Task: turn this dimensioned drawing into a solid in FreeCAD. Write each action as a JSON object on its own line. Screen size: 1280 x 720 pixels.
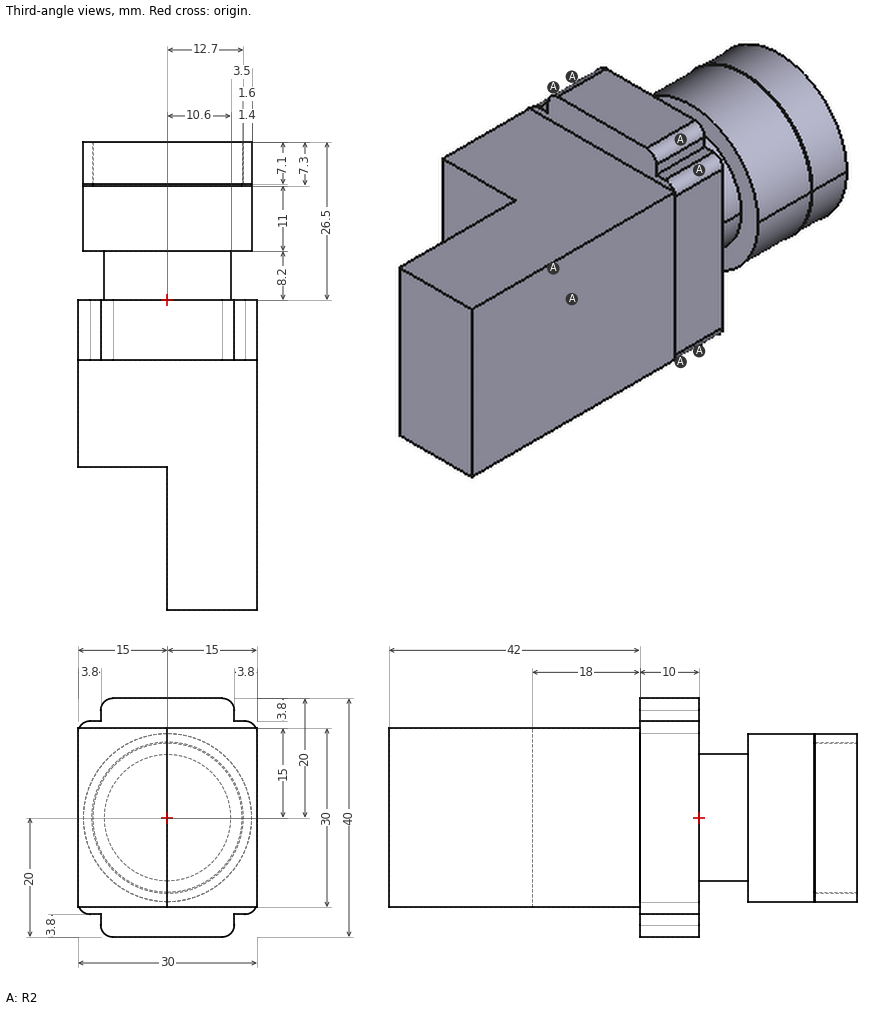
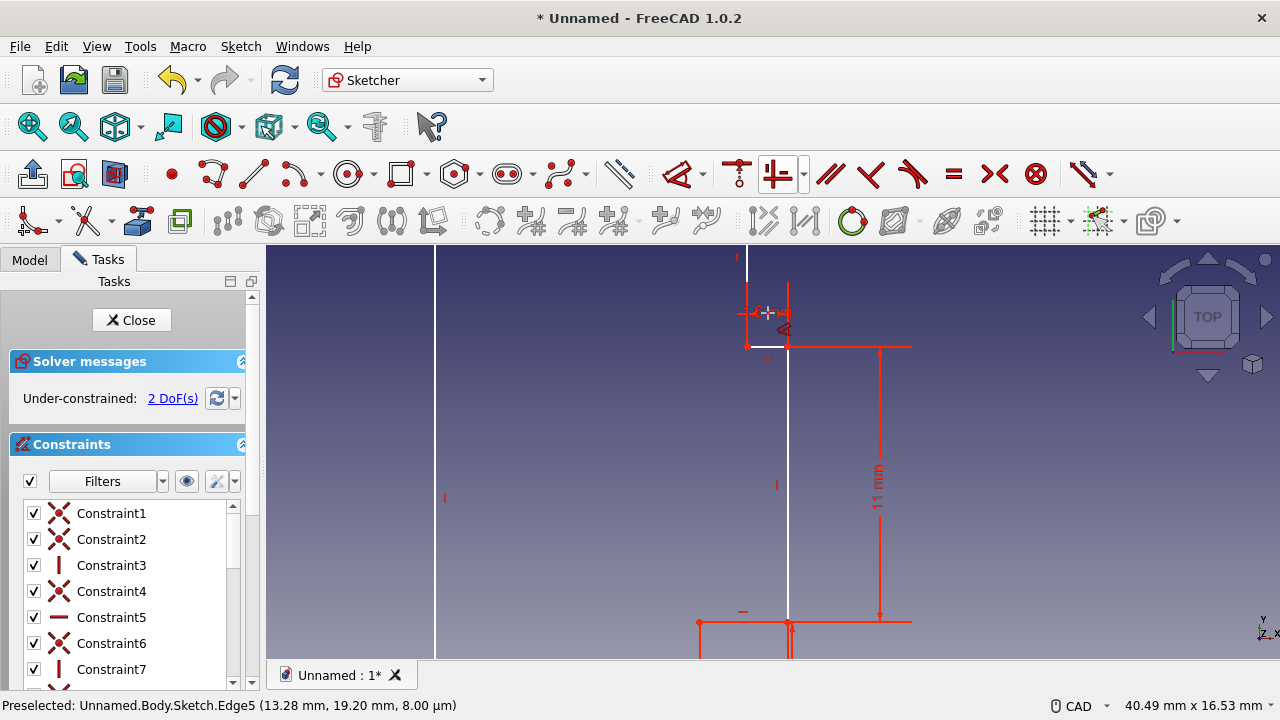
{"action": "left_click", "coordinate": [747, 293]}
{"action": "left_click", "coordinate": [781, 284]}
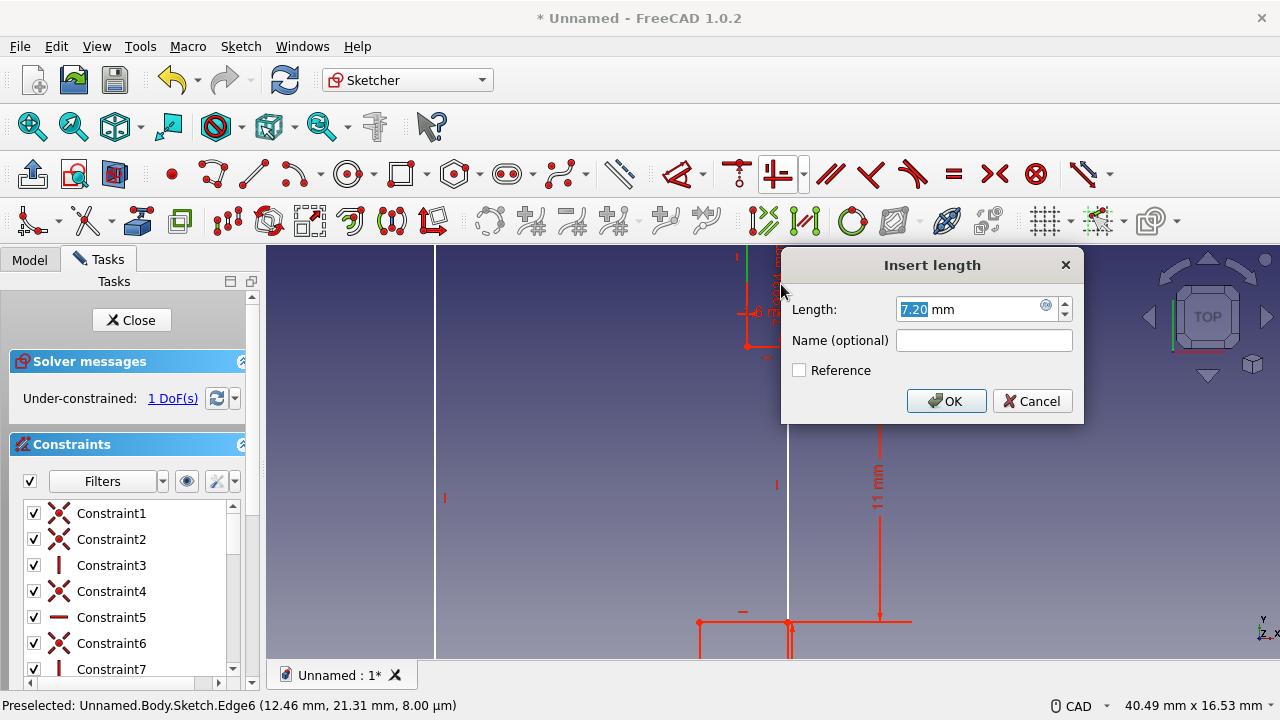
{"action": "type", "text": "7.3"}
{"action": "key", "text": "Return"}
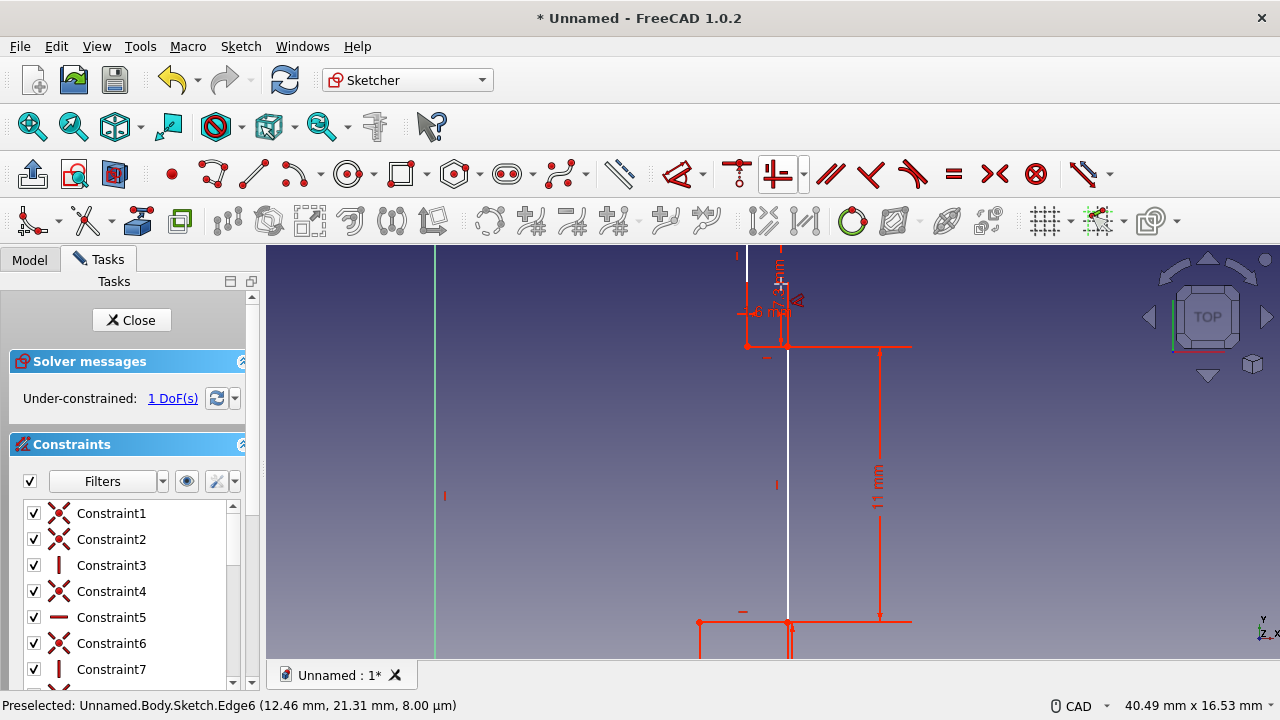
{"action": "scroll", "coordinate": [758, 426], "scroll_direction": "down", "scroll_amount": 5}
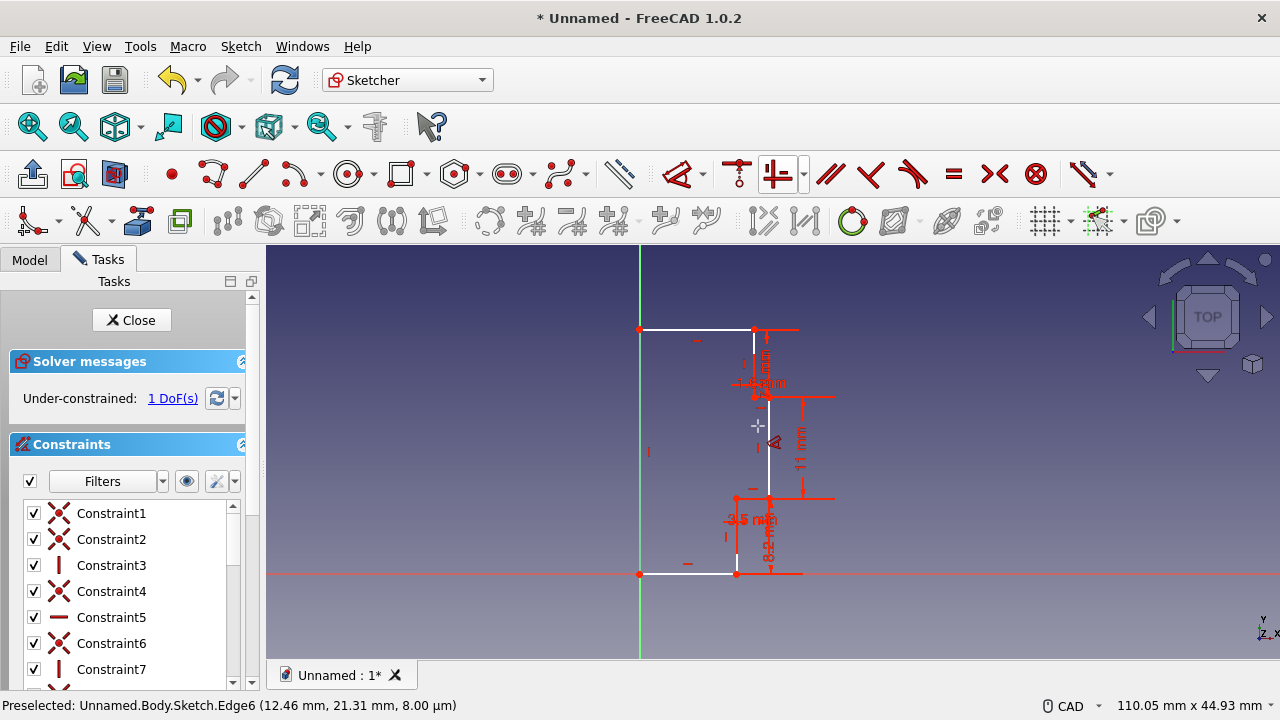
{"action": "left_click", "coordinate": [669, 574]}
{"action": "left_click", "coordinate": [688, 608]}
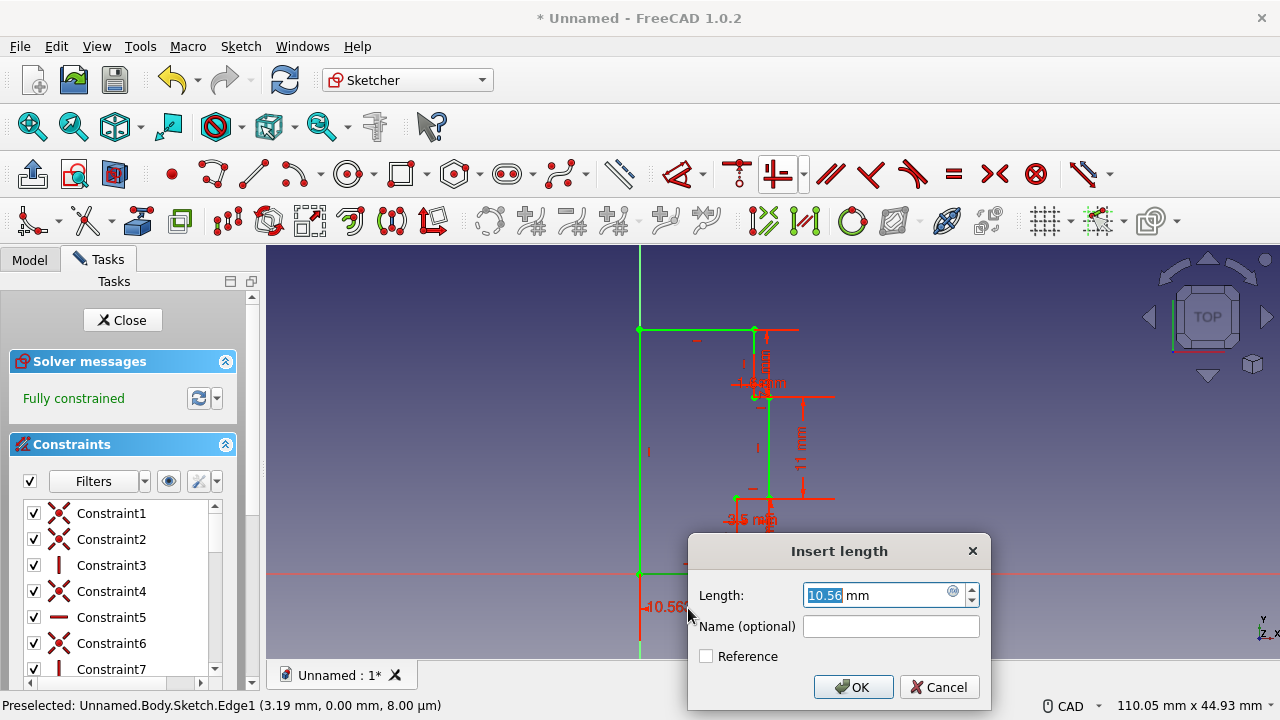
{"action": "type", "text": "10.6"}
{"action": "key", "text": "Return"}
{"action": "key", "text": "Escape"}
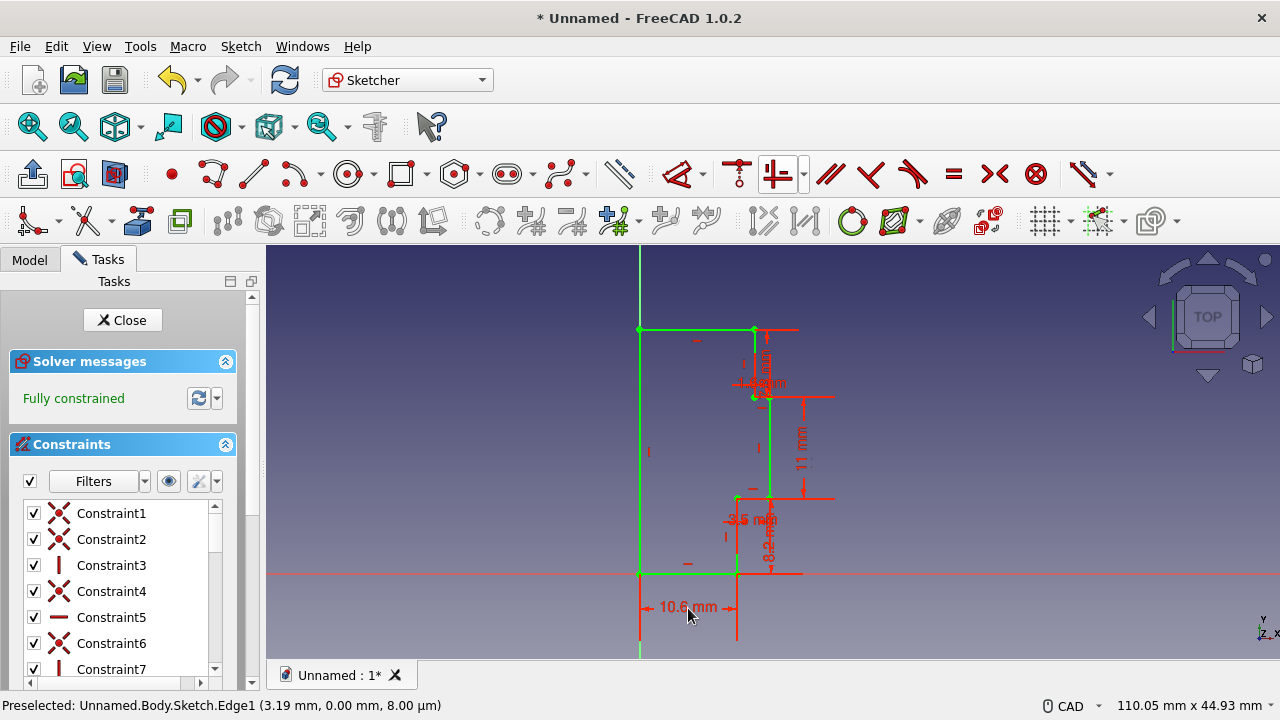
{"action": "left_click", "coordinate": [123, 320]}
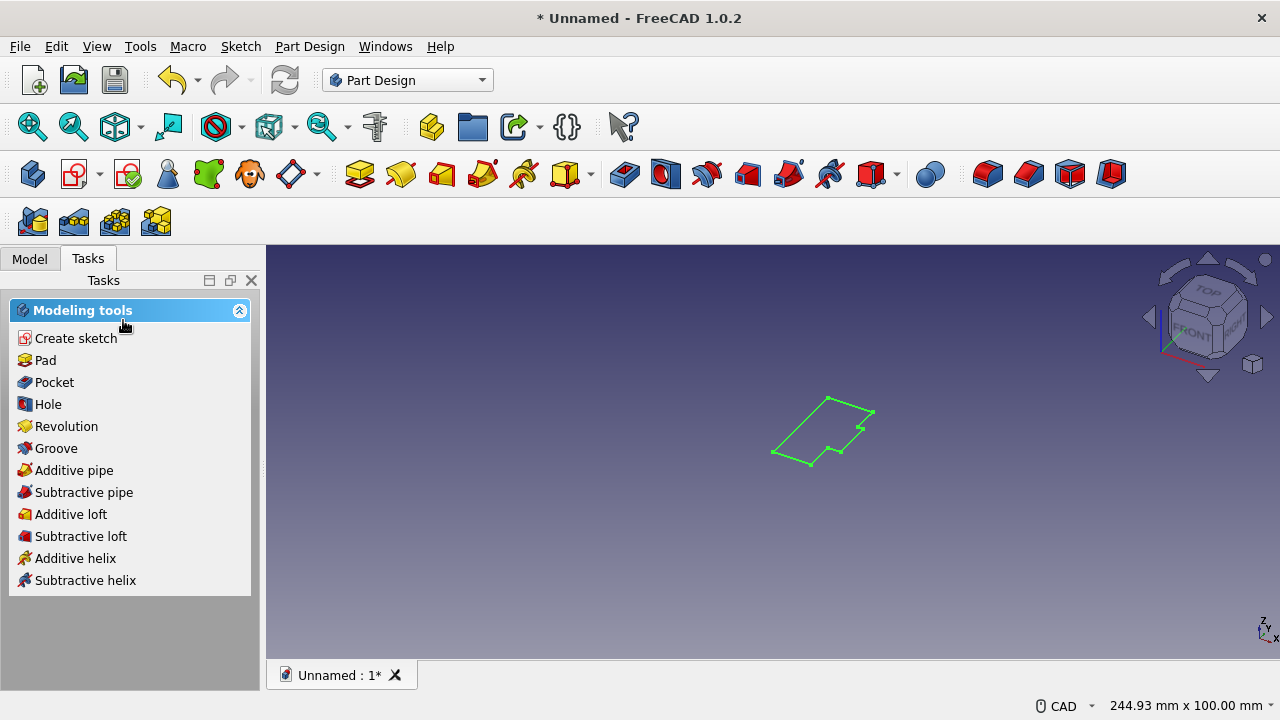
{"action": "left_click", "coordinate": [401, 174]}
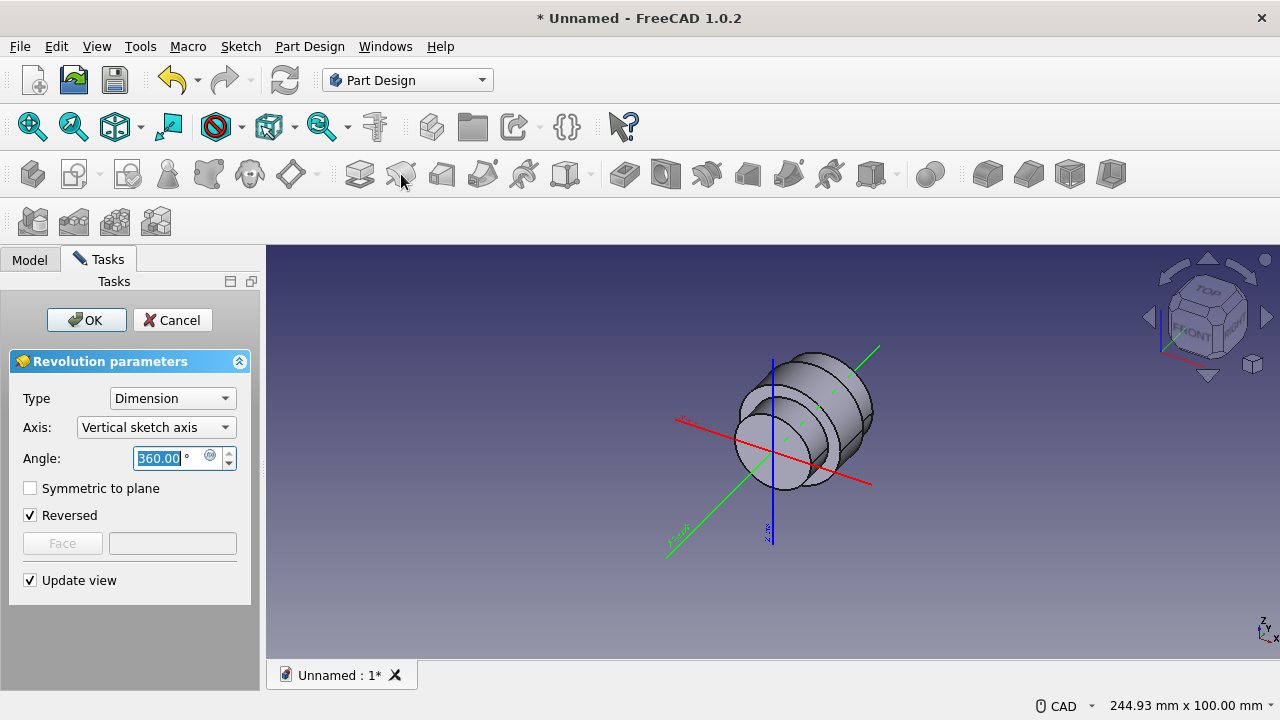
{"action": "left_click", "coordinate": [87, 320]}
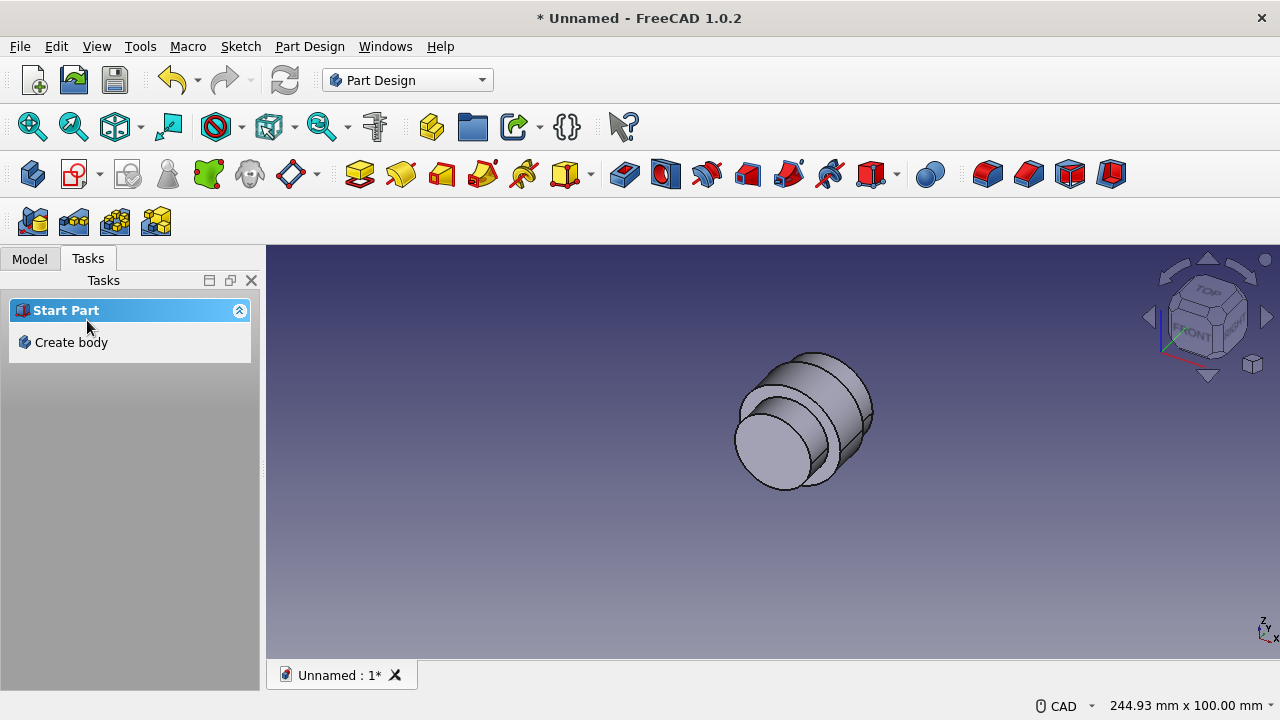
{"action": "key", "text": "v f"}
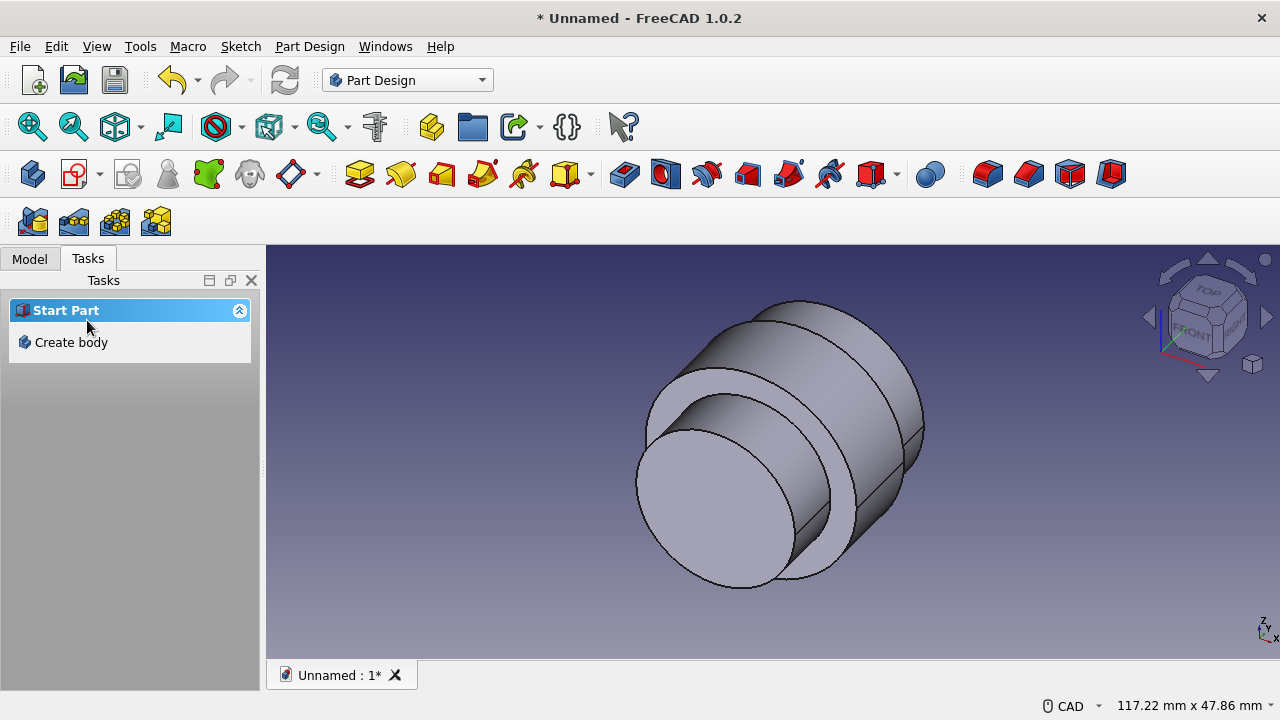
{"action": "left_click", "coordinate": [33, 174]}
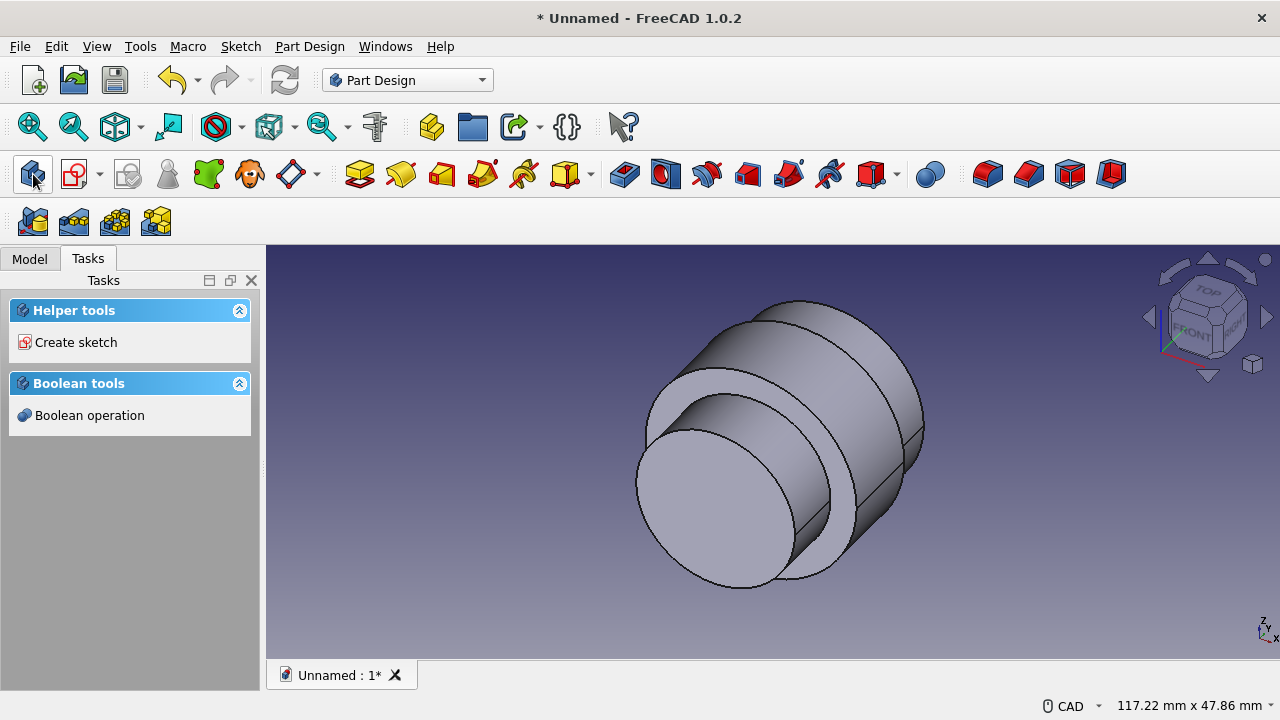
{"action": "left_click", "coordinate": [306, 619]}